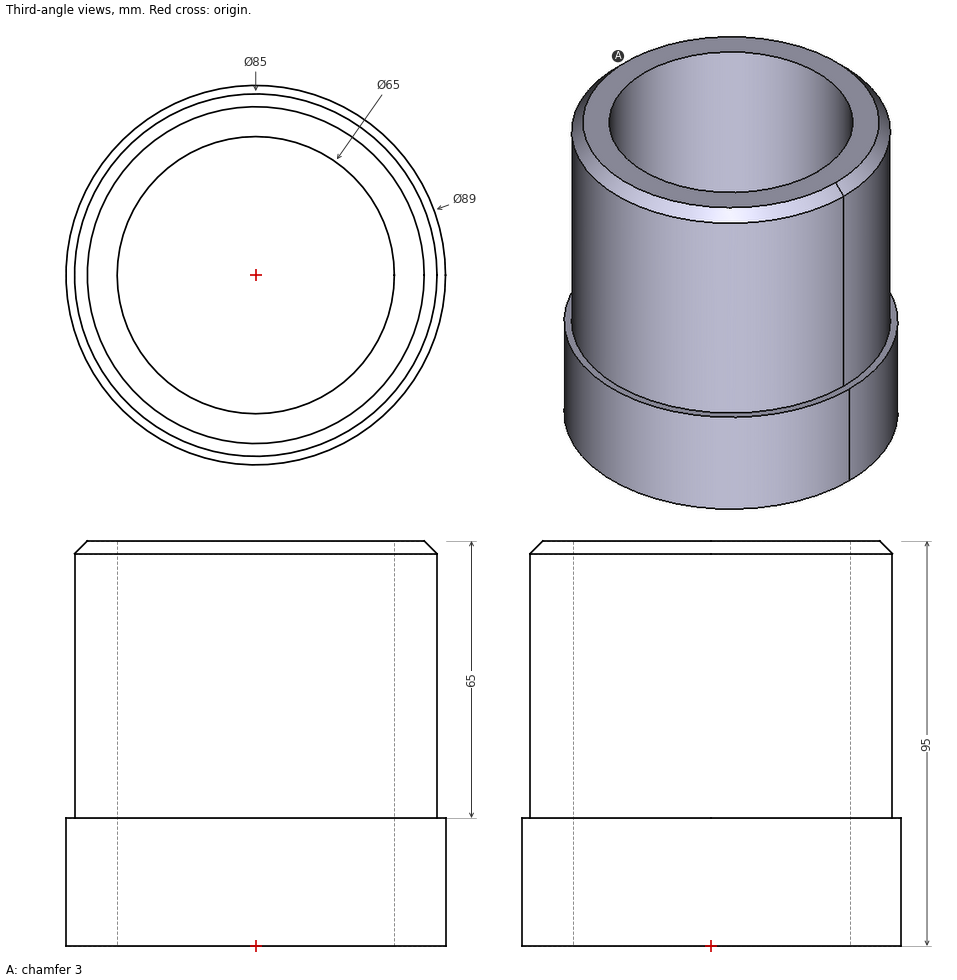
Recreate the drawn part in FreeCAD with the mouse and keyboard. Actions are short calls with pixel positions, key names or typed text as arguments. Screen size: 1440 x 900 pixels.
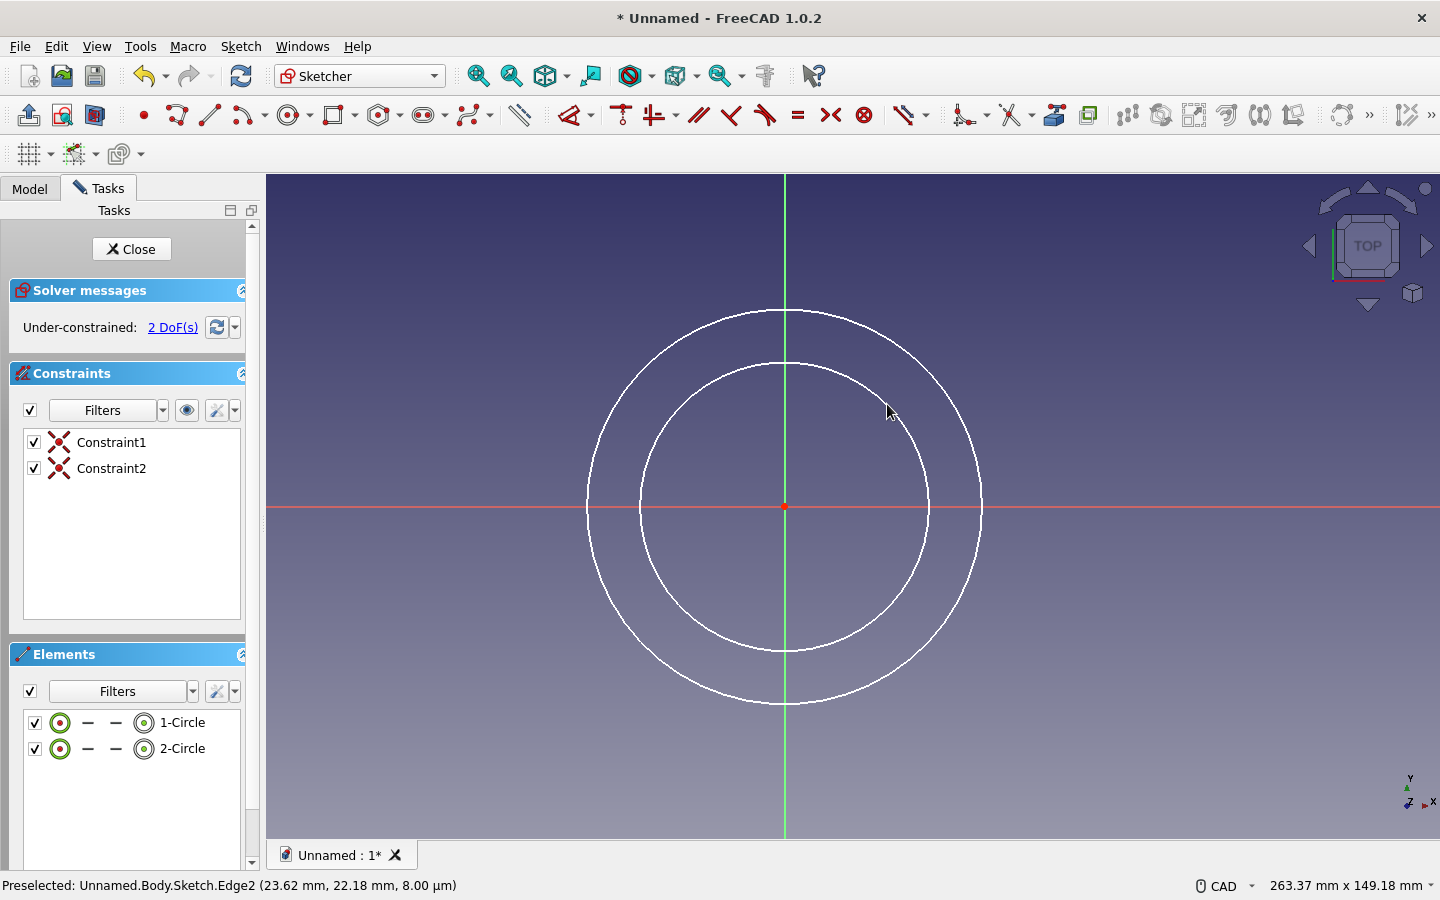
click(568, 116)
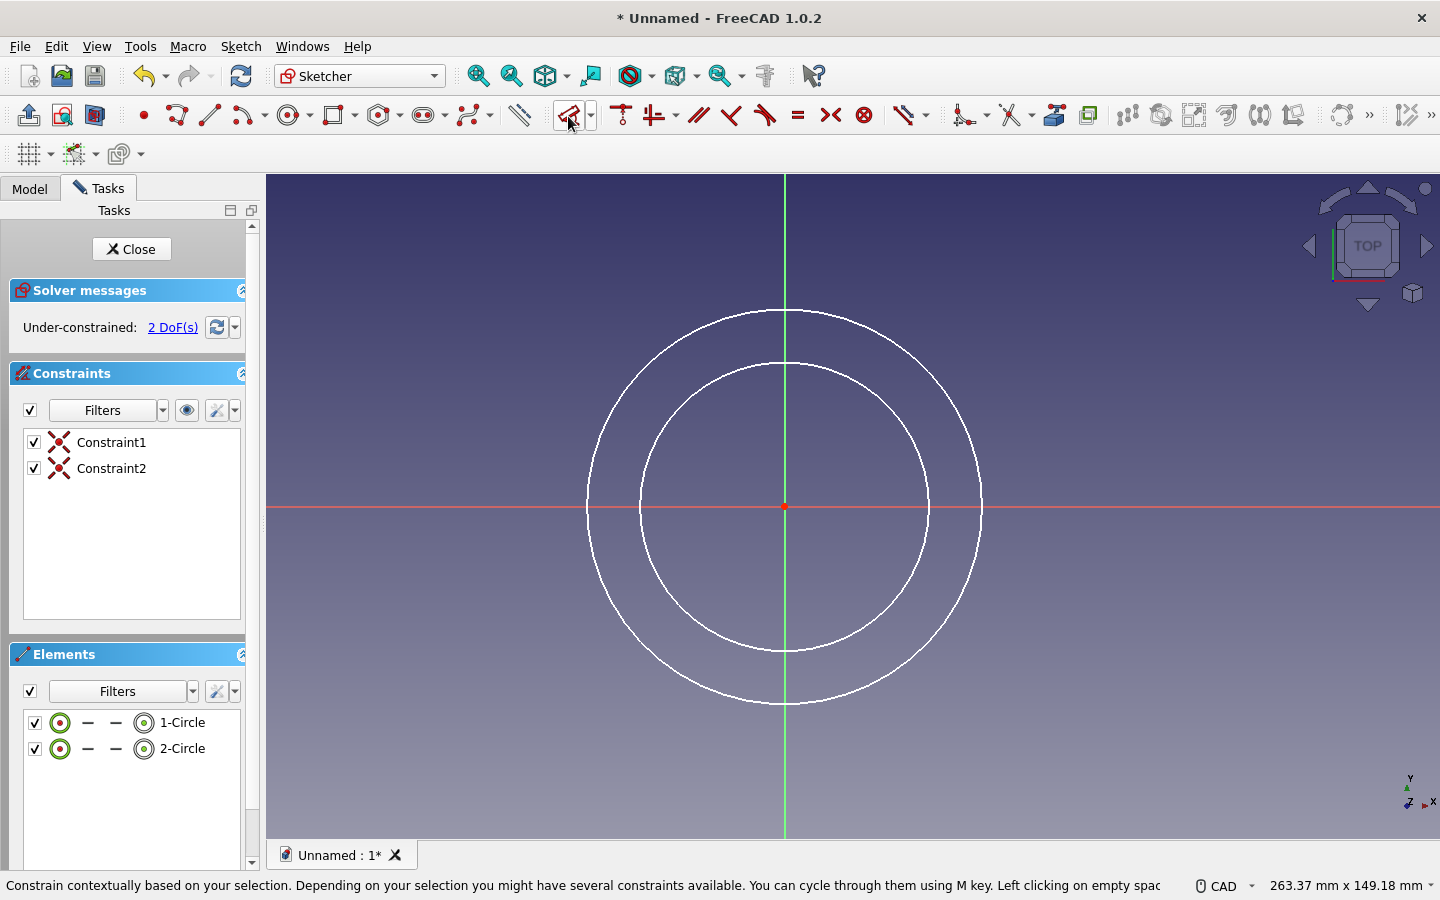
click(924, 367)
click(947, 344)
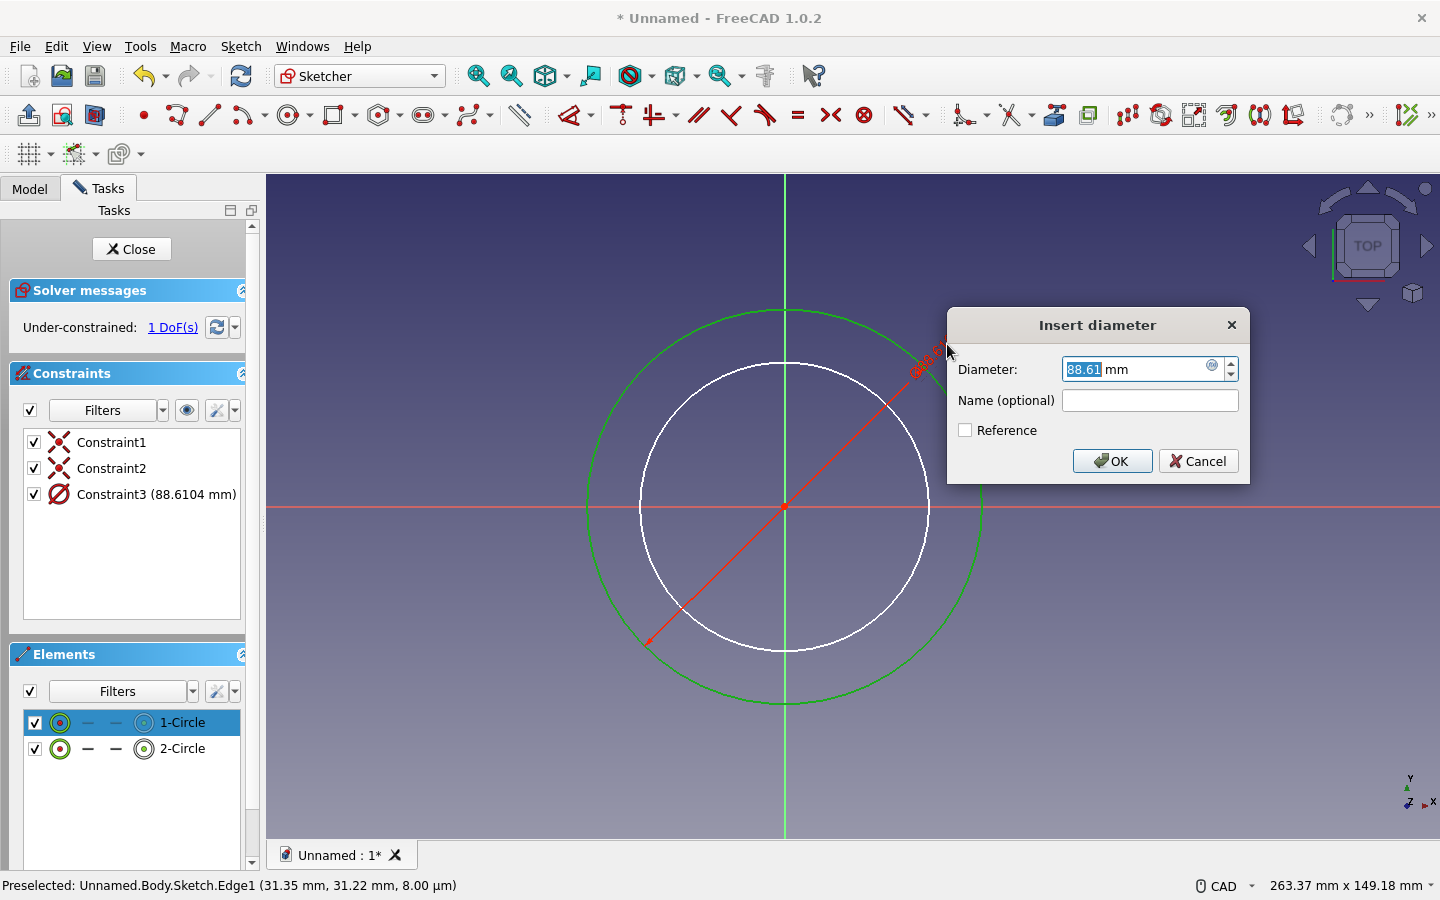
text(89)
key(Return)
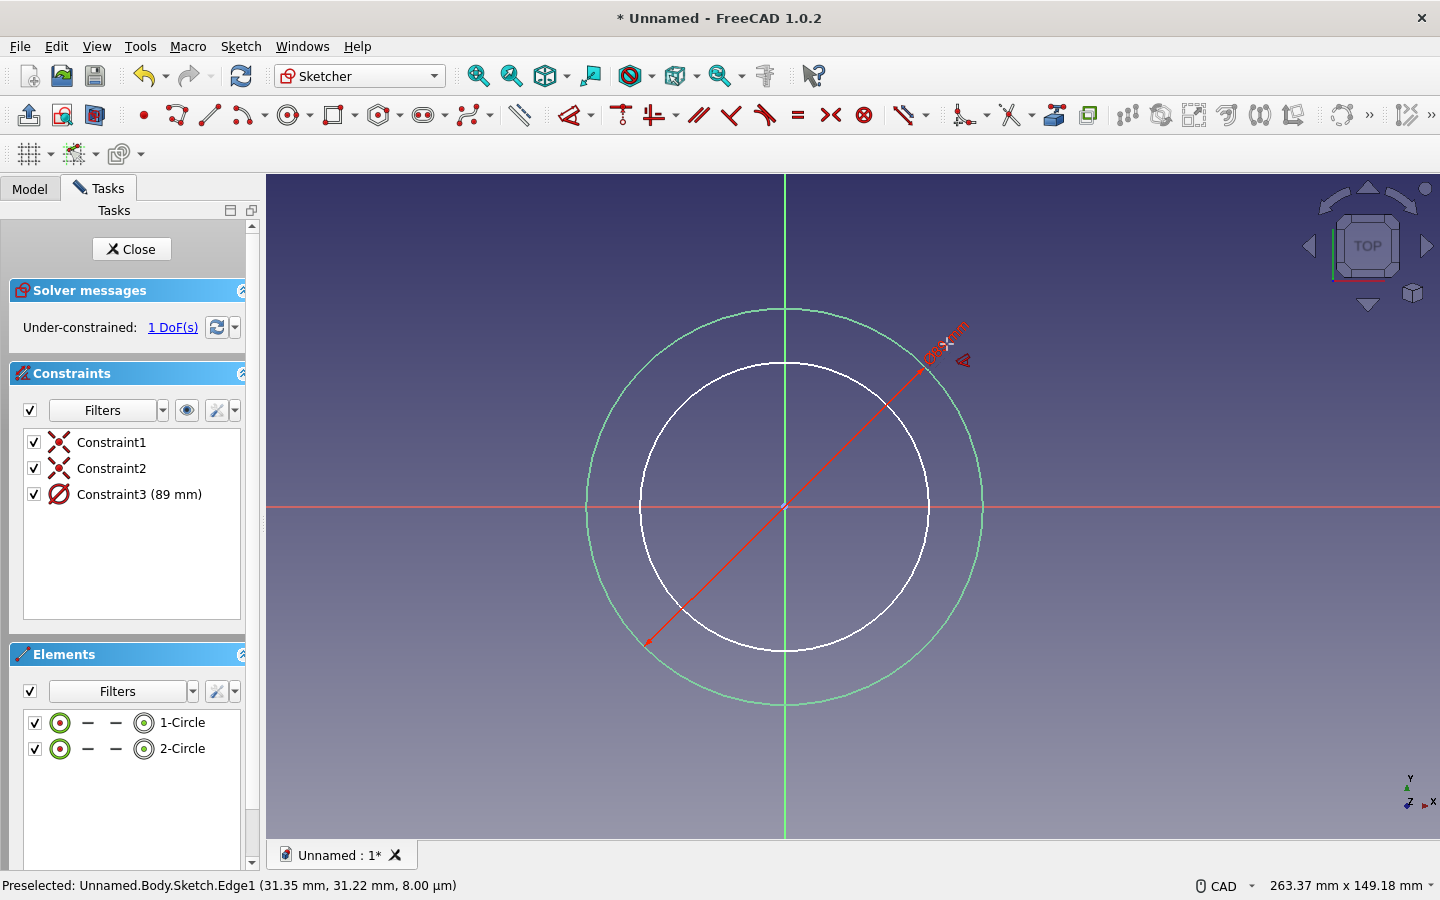
click(886, 404)
click(908, 381)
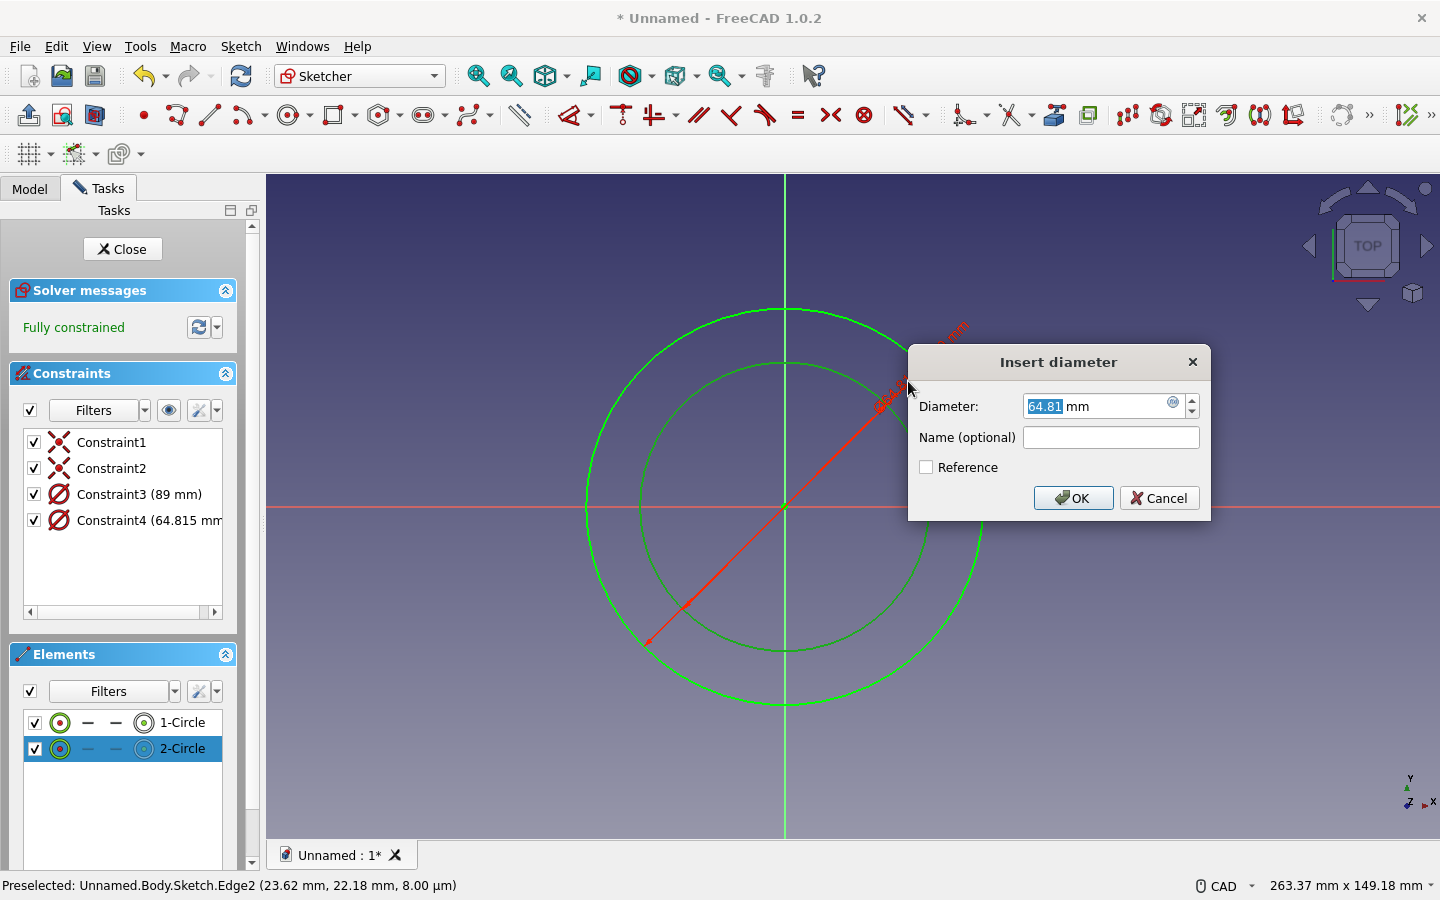
text(65)
key(Return)
key(Escape)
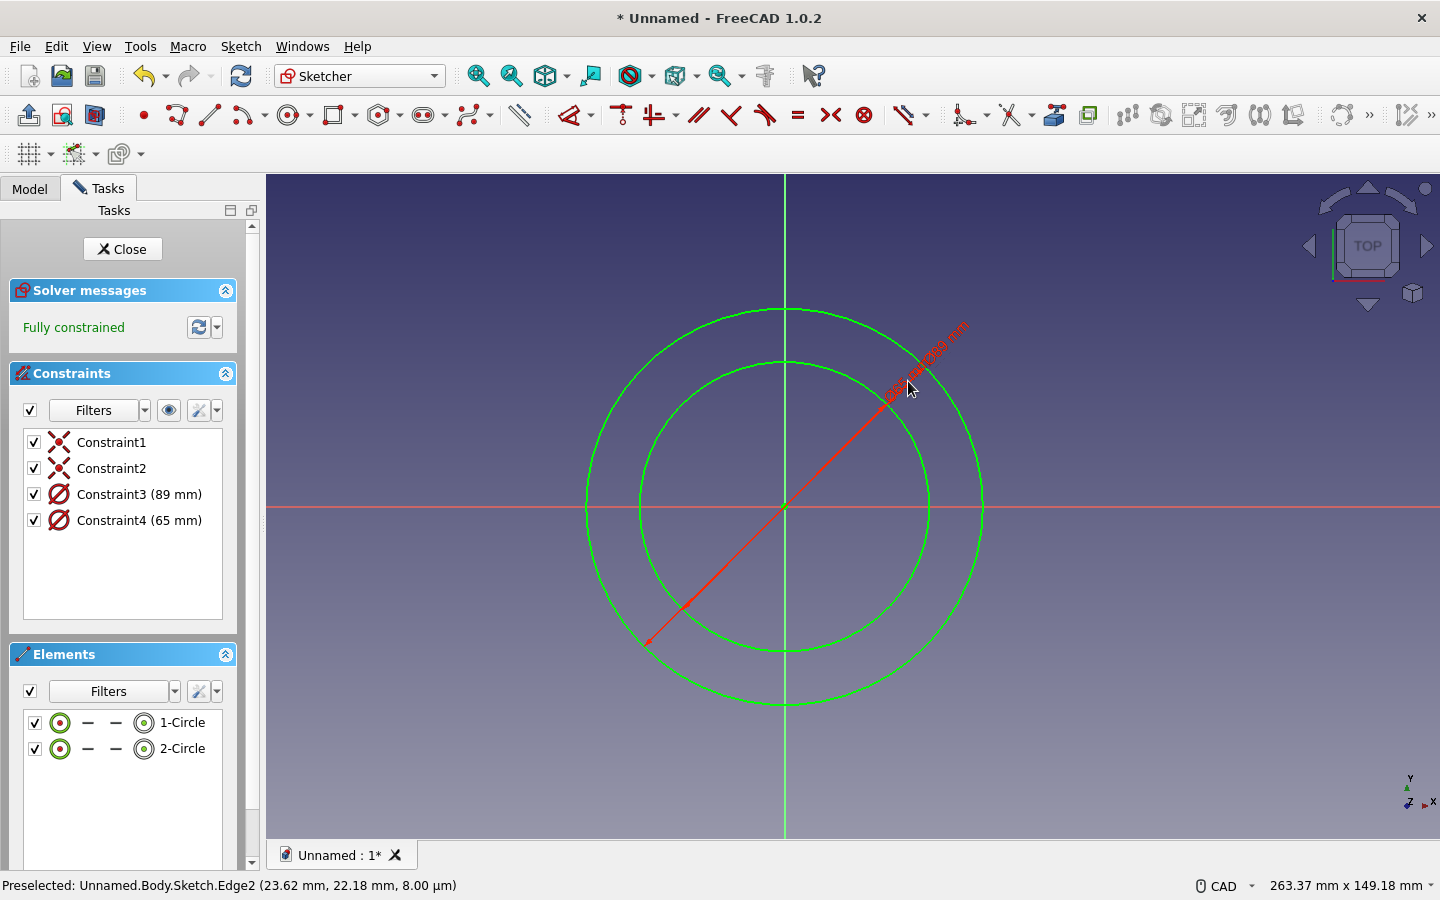
click(123, 249)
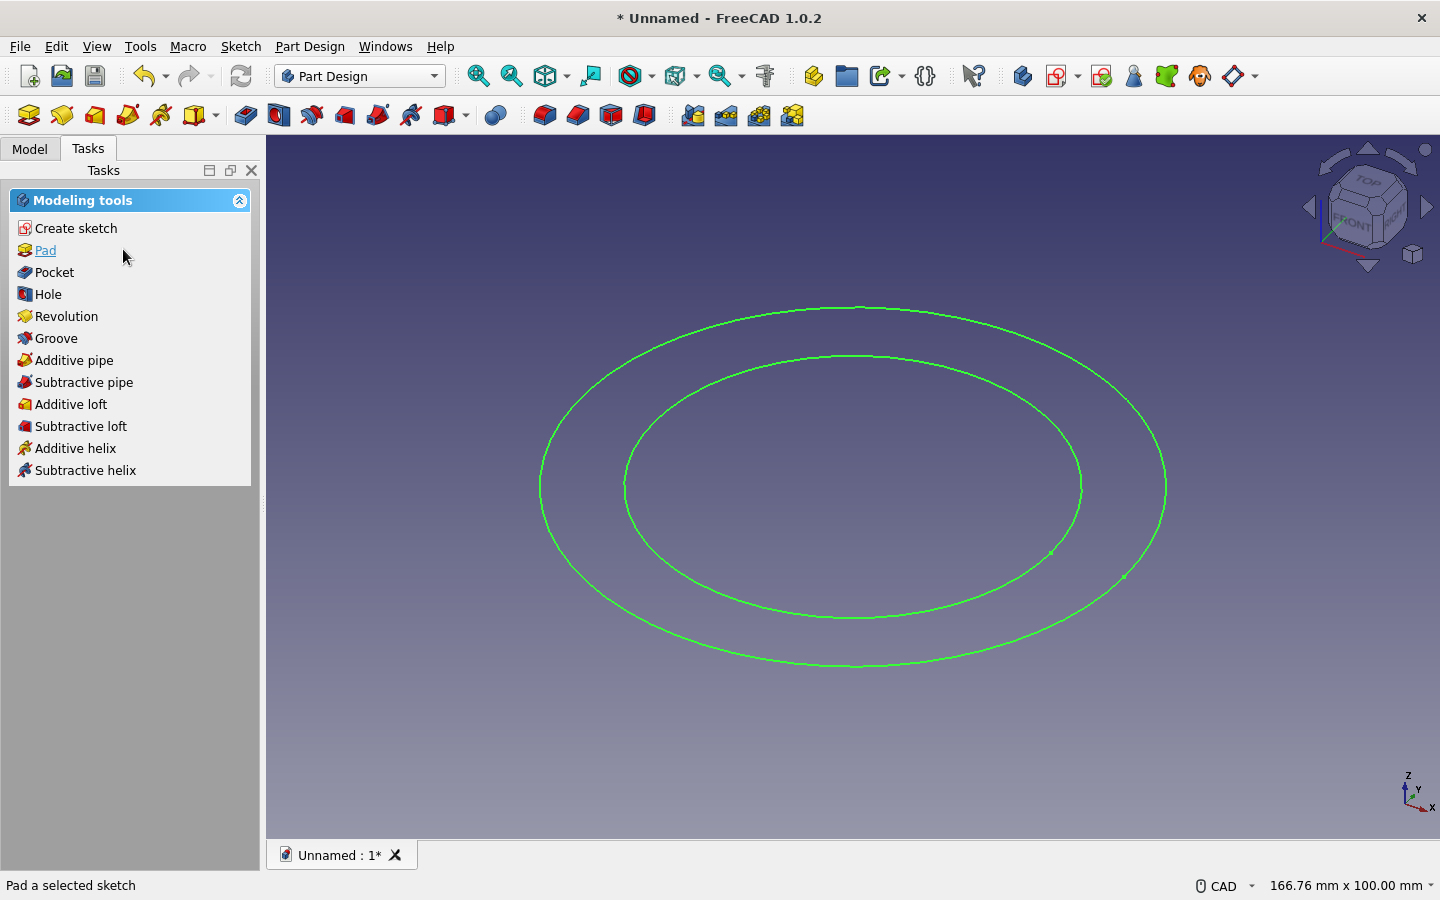
click(29, 116)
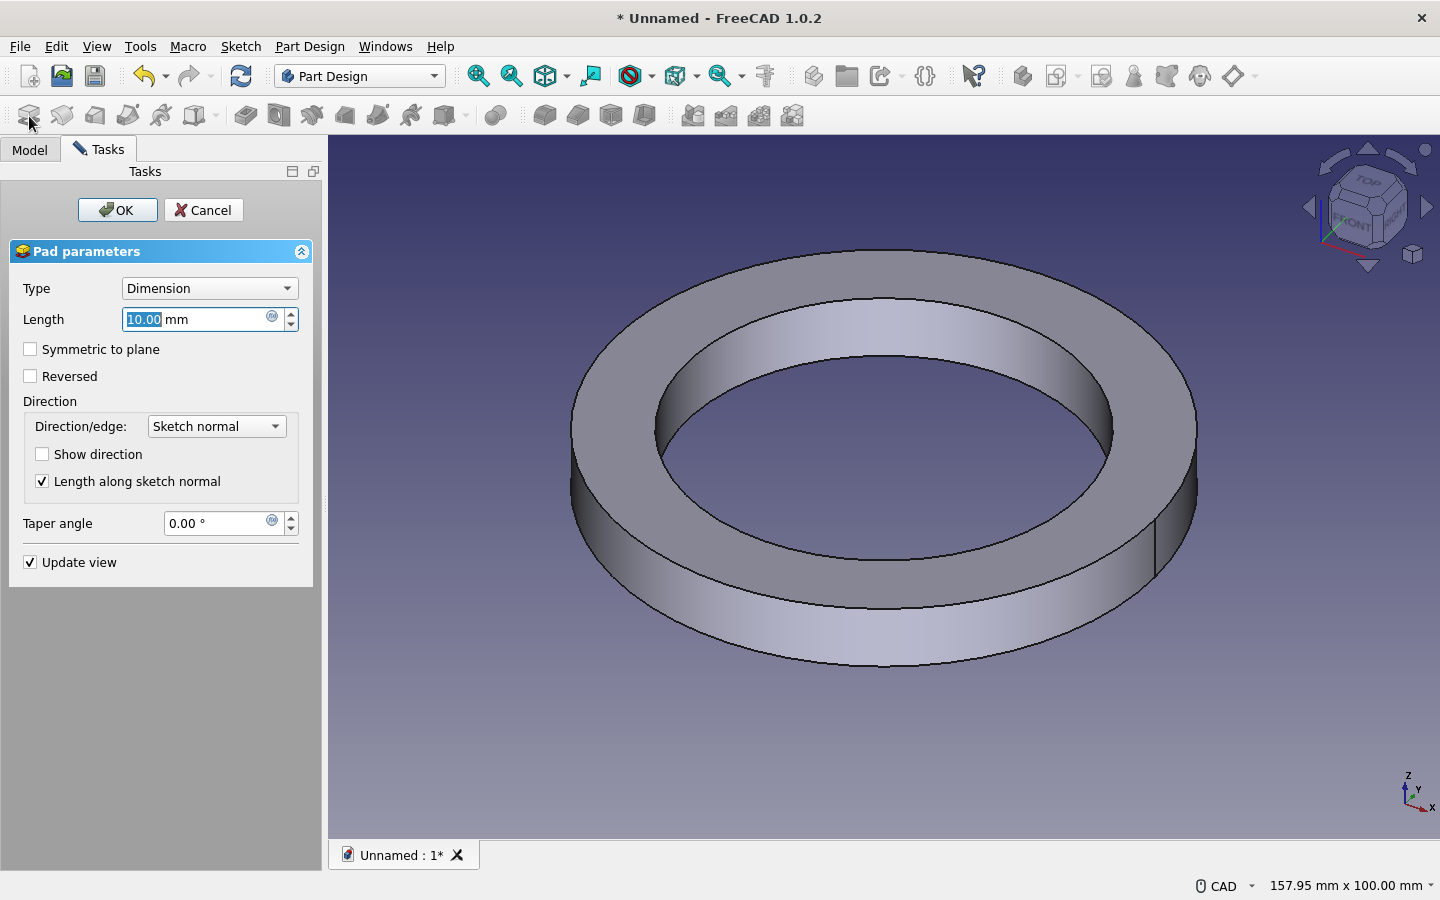
text(95)
key(Tab)